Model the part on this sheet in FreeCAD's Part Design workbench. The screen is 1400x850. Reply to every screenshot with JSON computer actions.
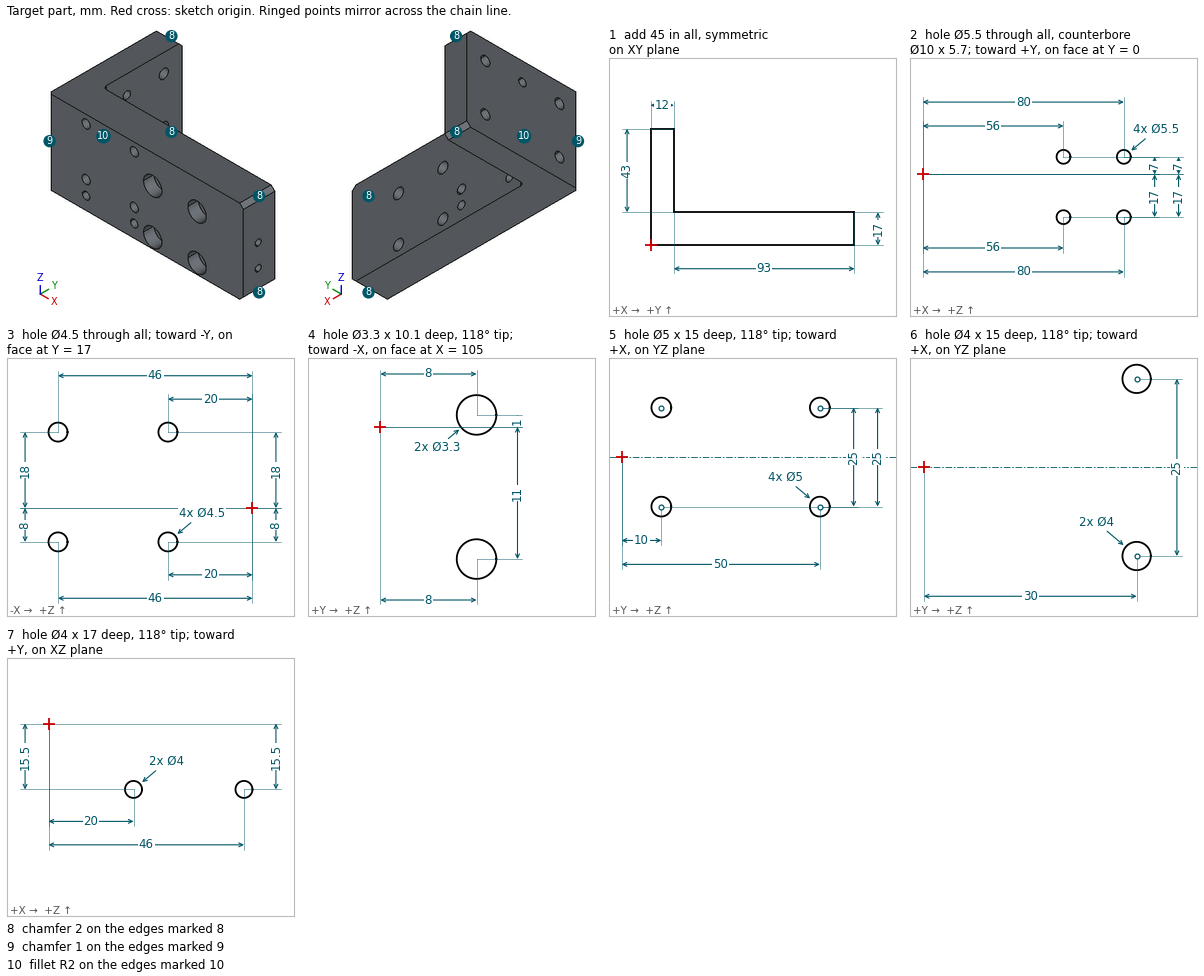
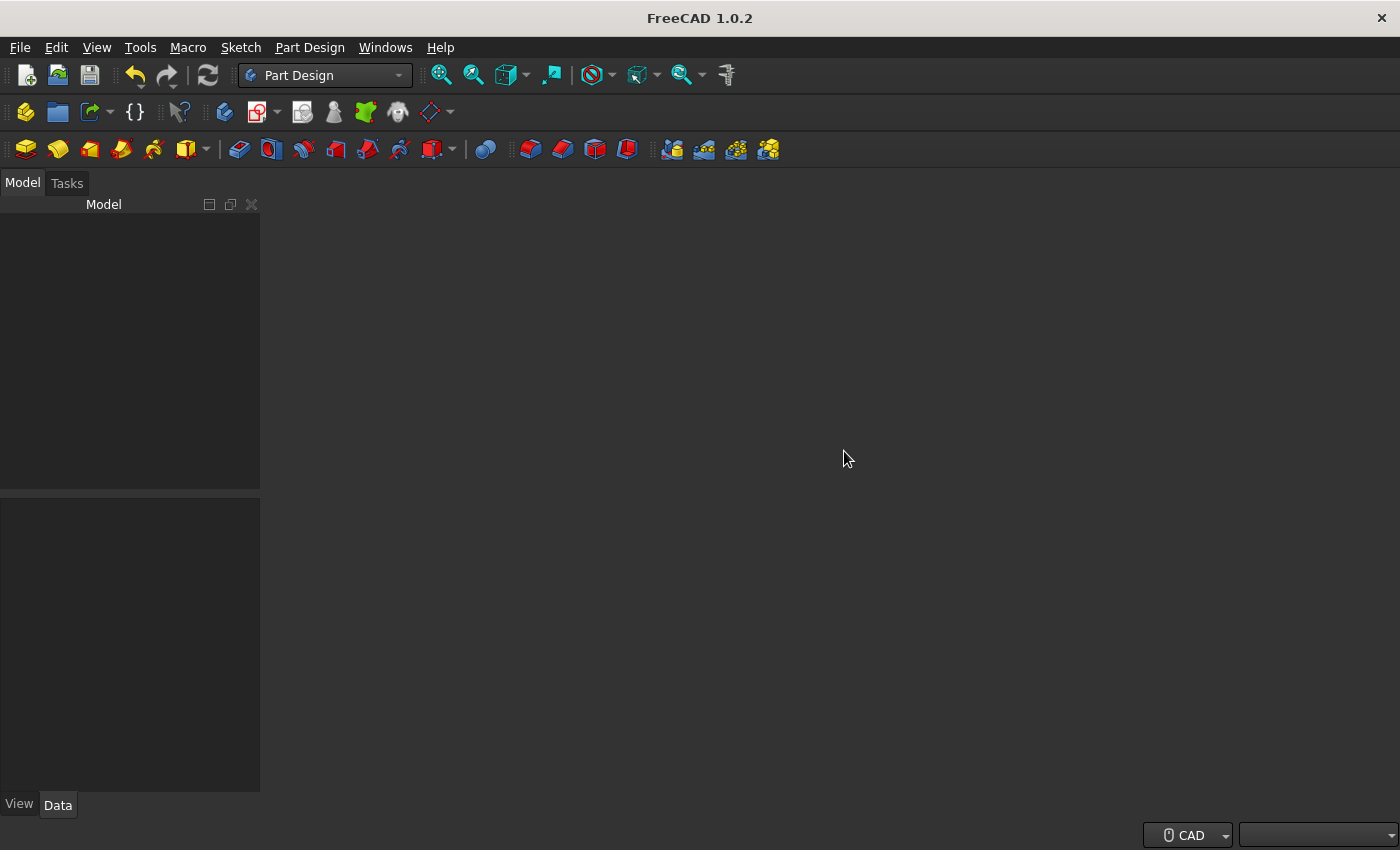
{"action": "key", "text": "ctrl+n"}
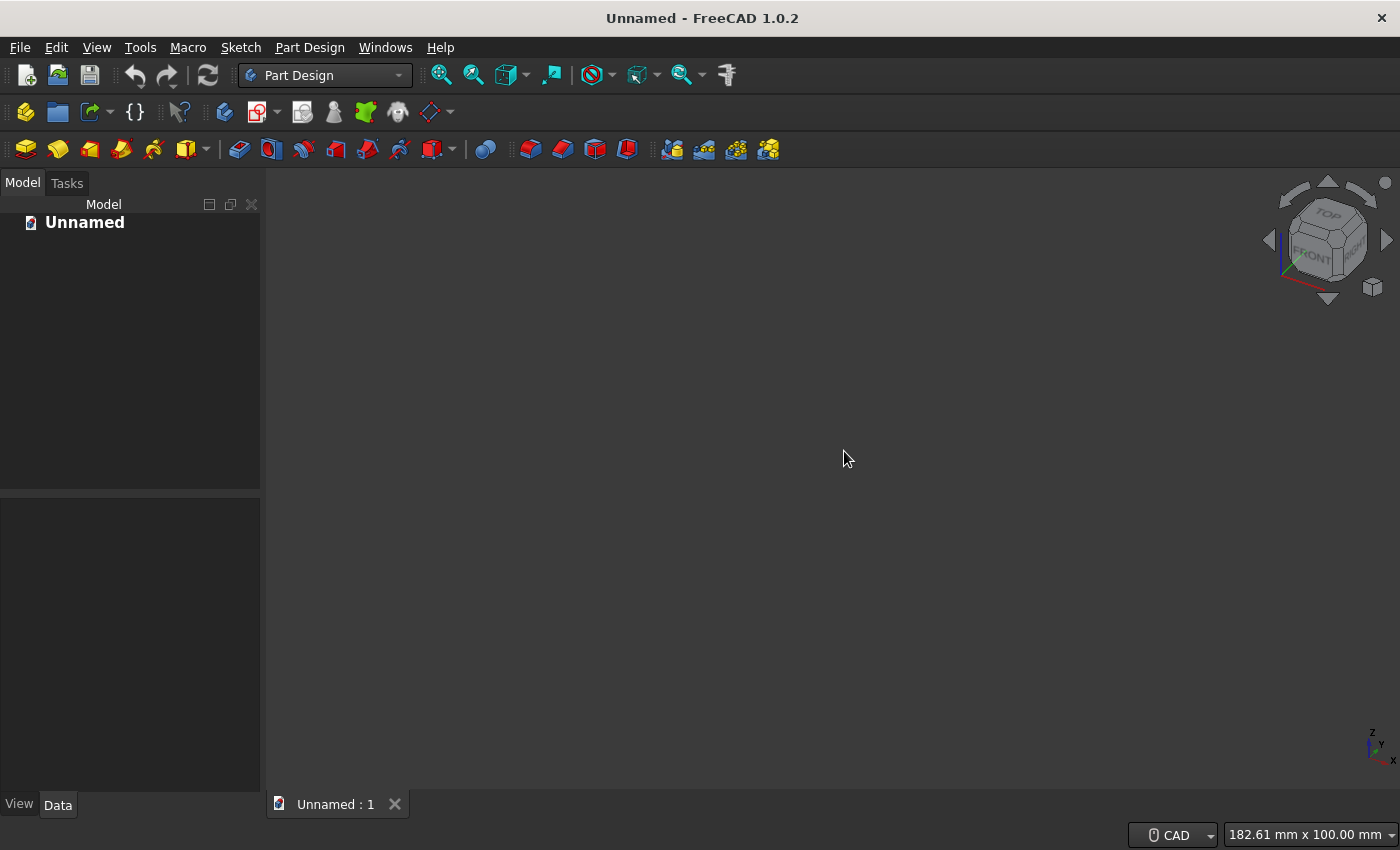
{"action": "left_click", "coordinate": [258, 112]}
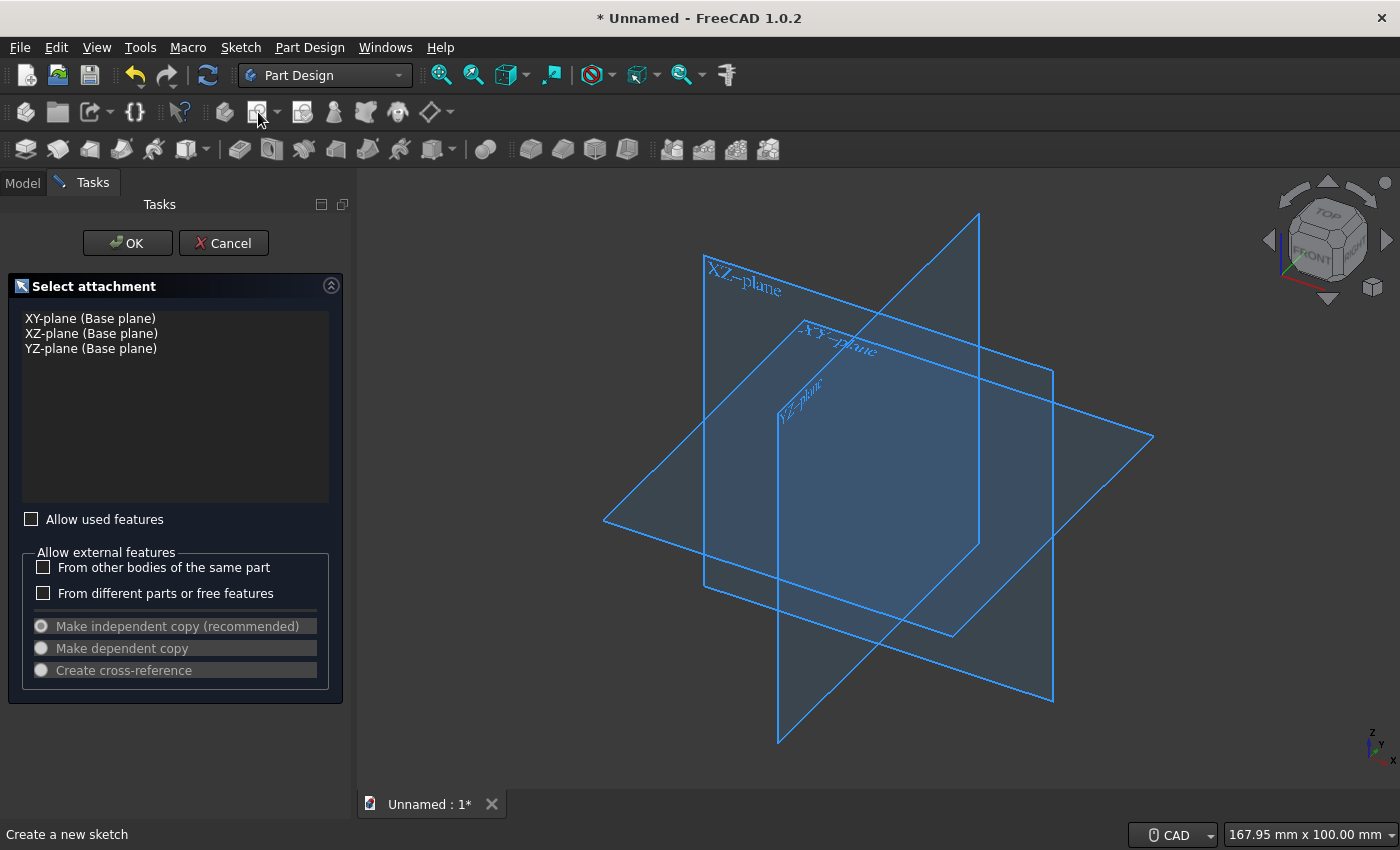
{"action": "left_click", "coordinate": [82, 318]}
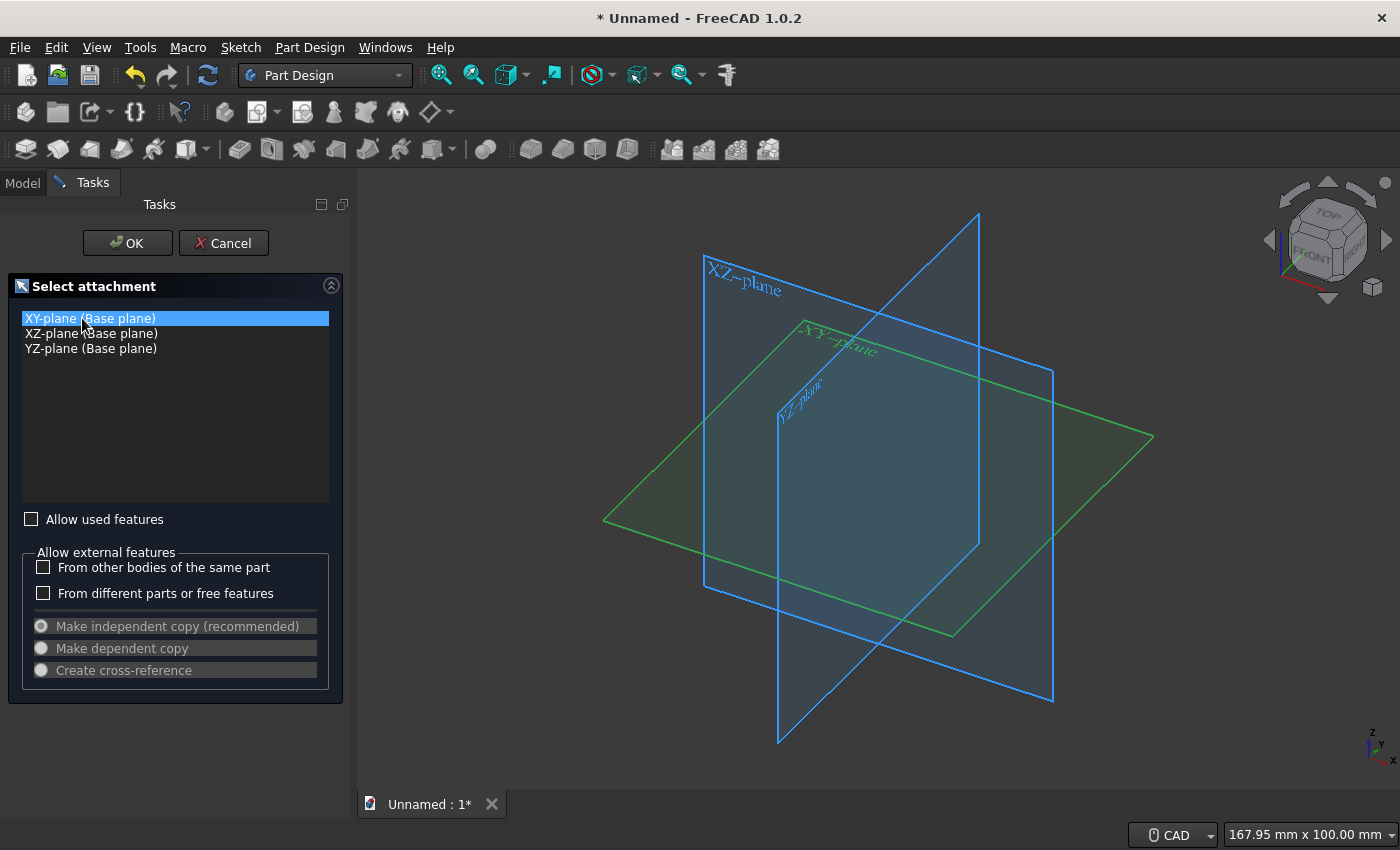
{"action": "left_click", "coordinate": [128, 243]}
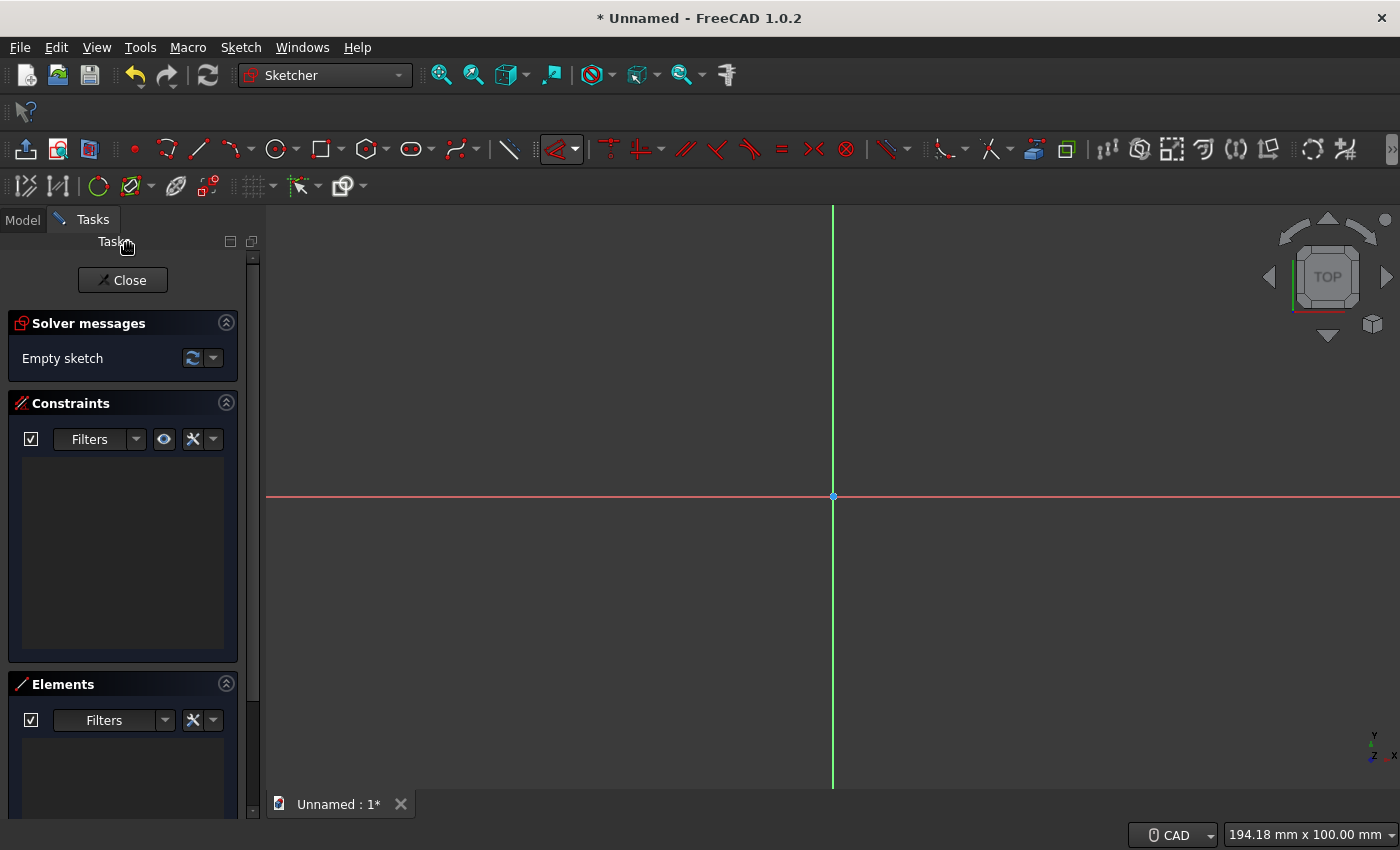
{"action": "scroll", "coordinate": [294, 761], "scroll_direction": "down", "scroll_amount": 2}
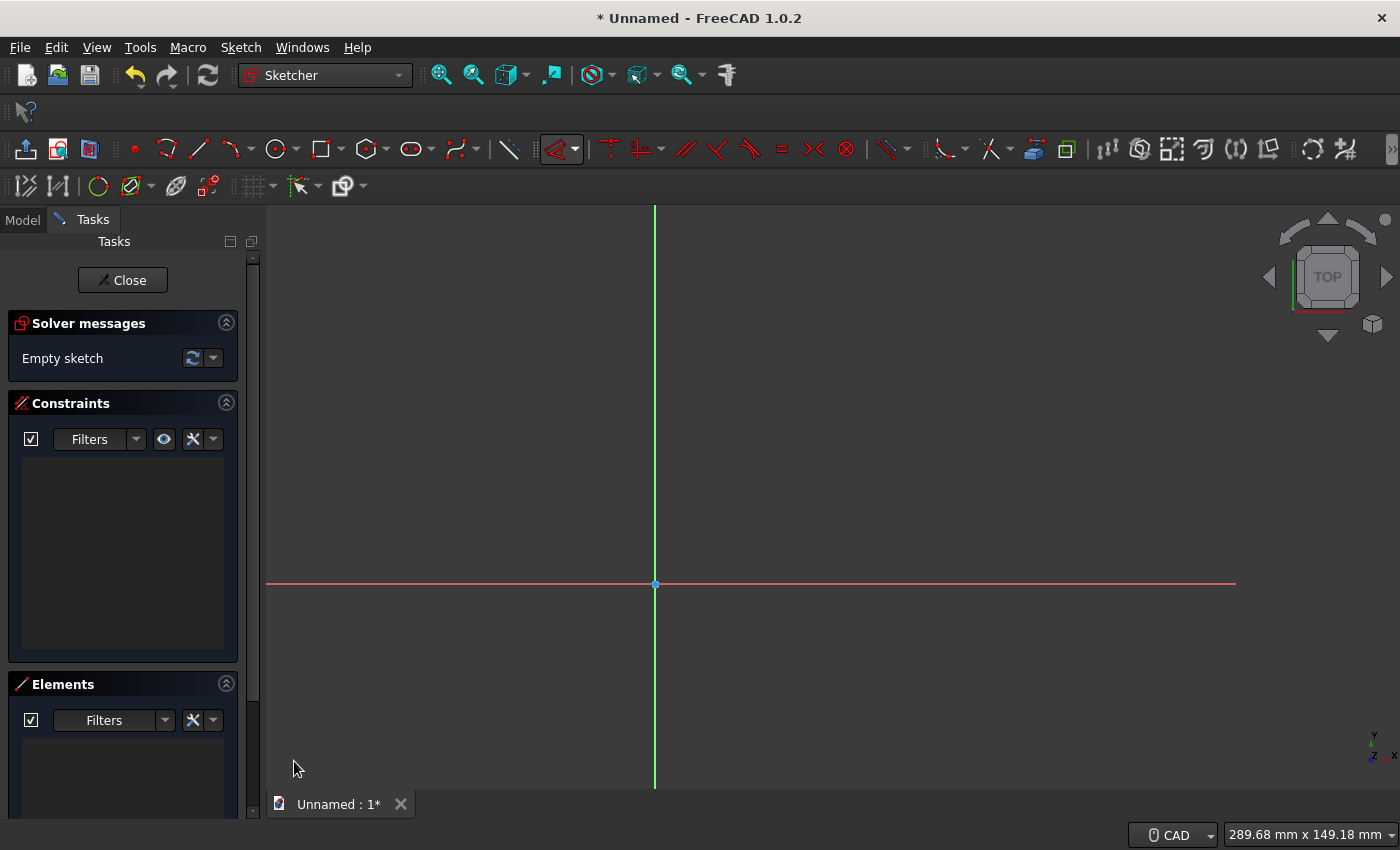
{"action": "scroll", "coordinate": [1057, 406], "scroll_direction": "up", "scroll_amount": 2}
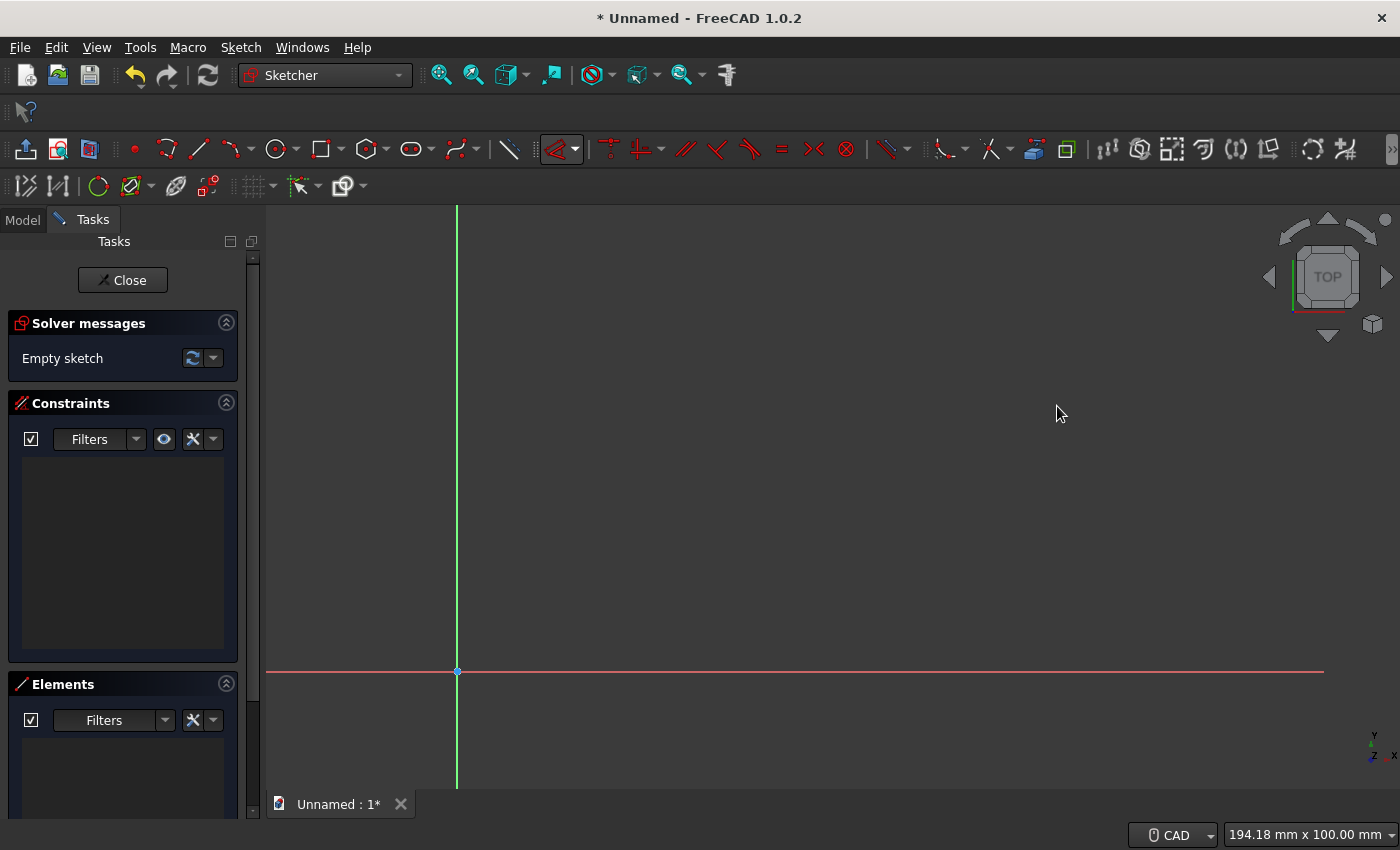
{"action": "left_click", "coordinate": [168, 150]}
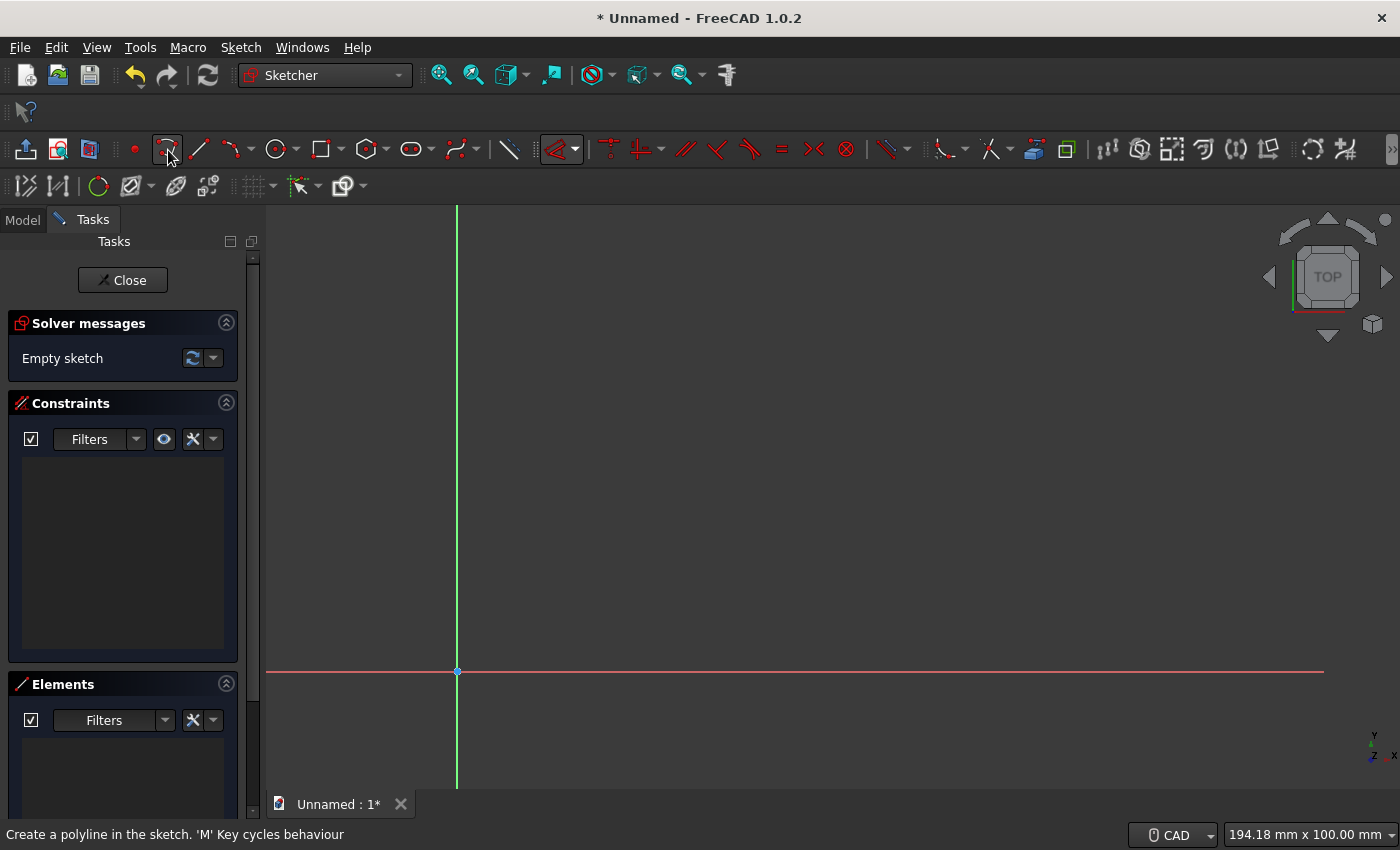
{"action": "left_click", "coordinate": [457, 672]}
{"action": "left_click", "coordinate": [1071, 663]}
{"action": "left_click", "coordinate": [1071, 573]}
{"action": "left_click", "coordinate": [527, 573]}
{"action": "left_click", "coordinate": [527, 321]}
{"action": "left_click", "coordinate": [466, 321]}
{"action": "left_click", "coordinate": [457, 672]}
{"action": "key", "text": "Escape"}
{"action": "key", "text": "Escape"}